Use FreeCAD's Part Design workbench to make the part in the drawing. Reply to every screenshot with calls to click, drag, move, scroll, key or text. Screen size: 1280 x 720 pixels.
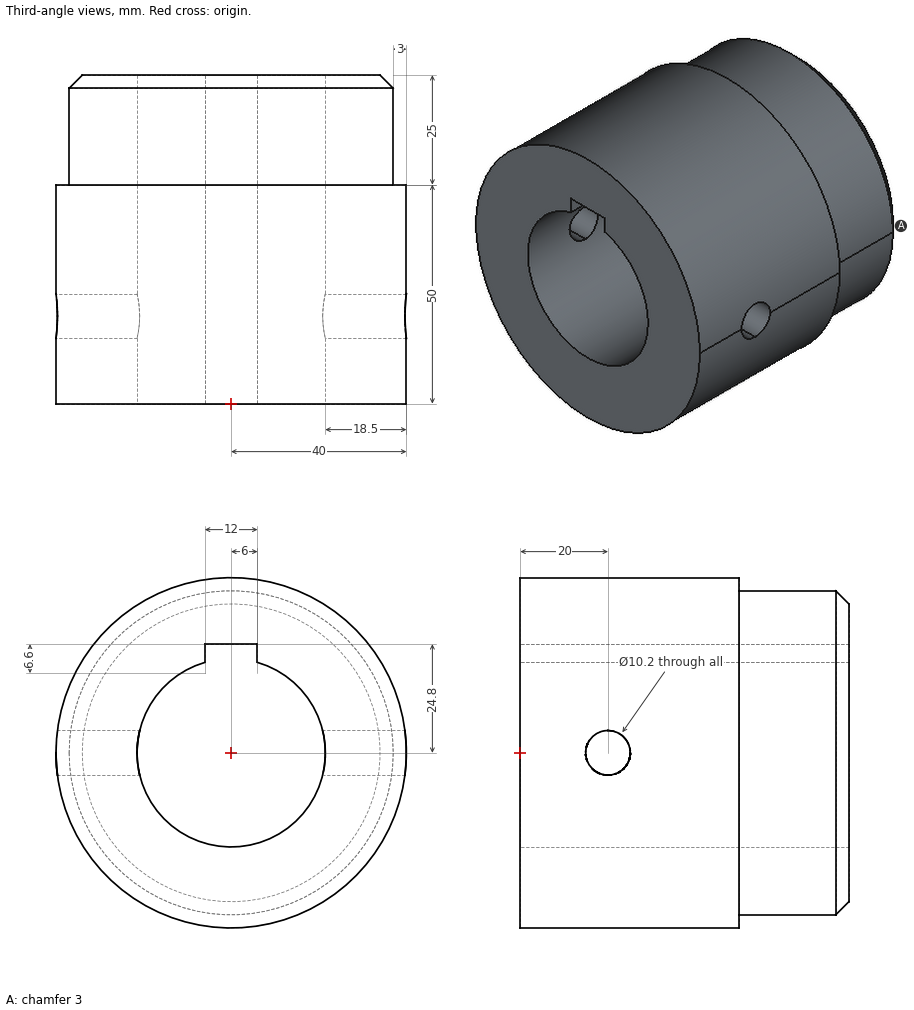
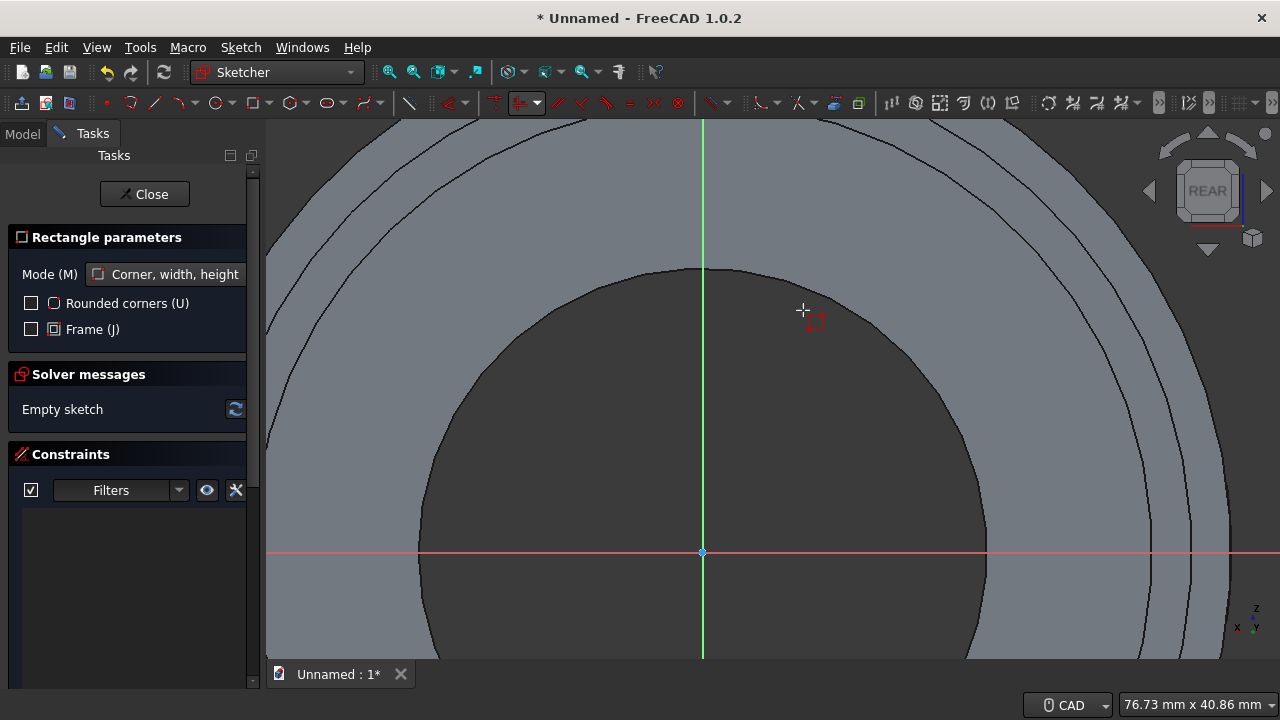
click(623, 225)
move(782, 312)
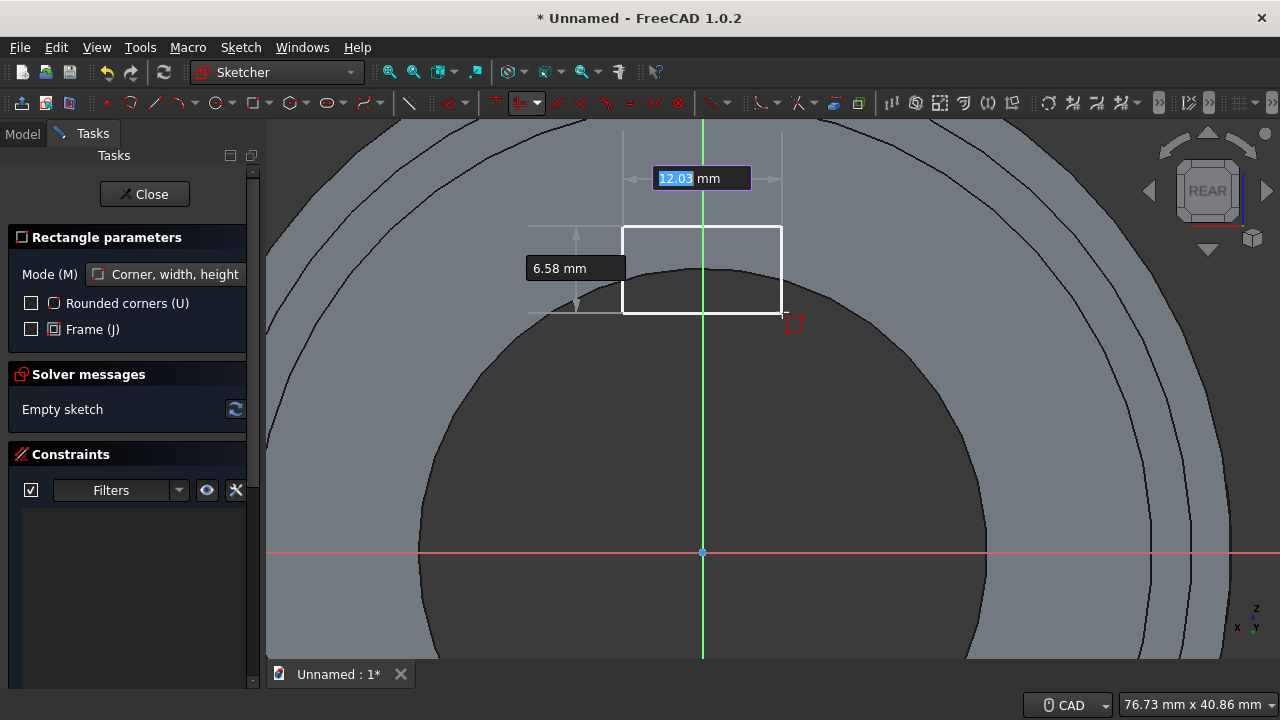
text(12)
key(Tab)
text(6.6)
key(Return)
key(Escape)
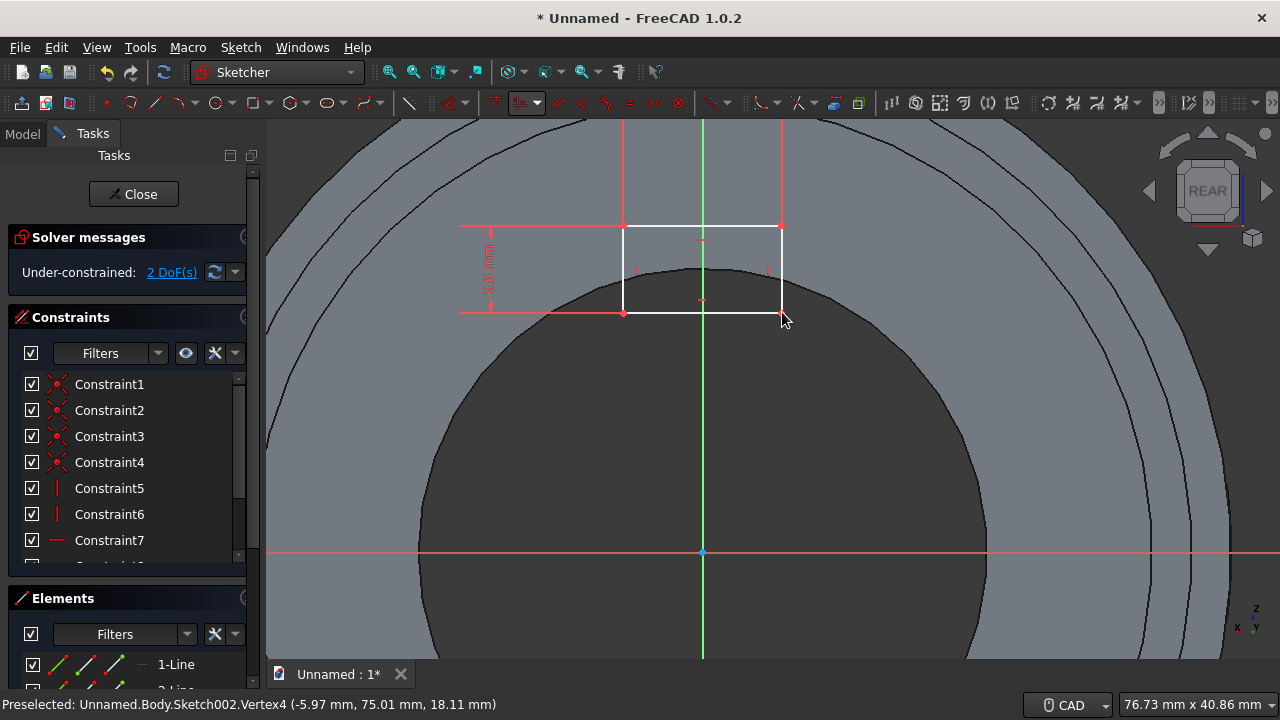
click(448, 104)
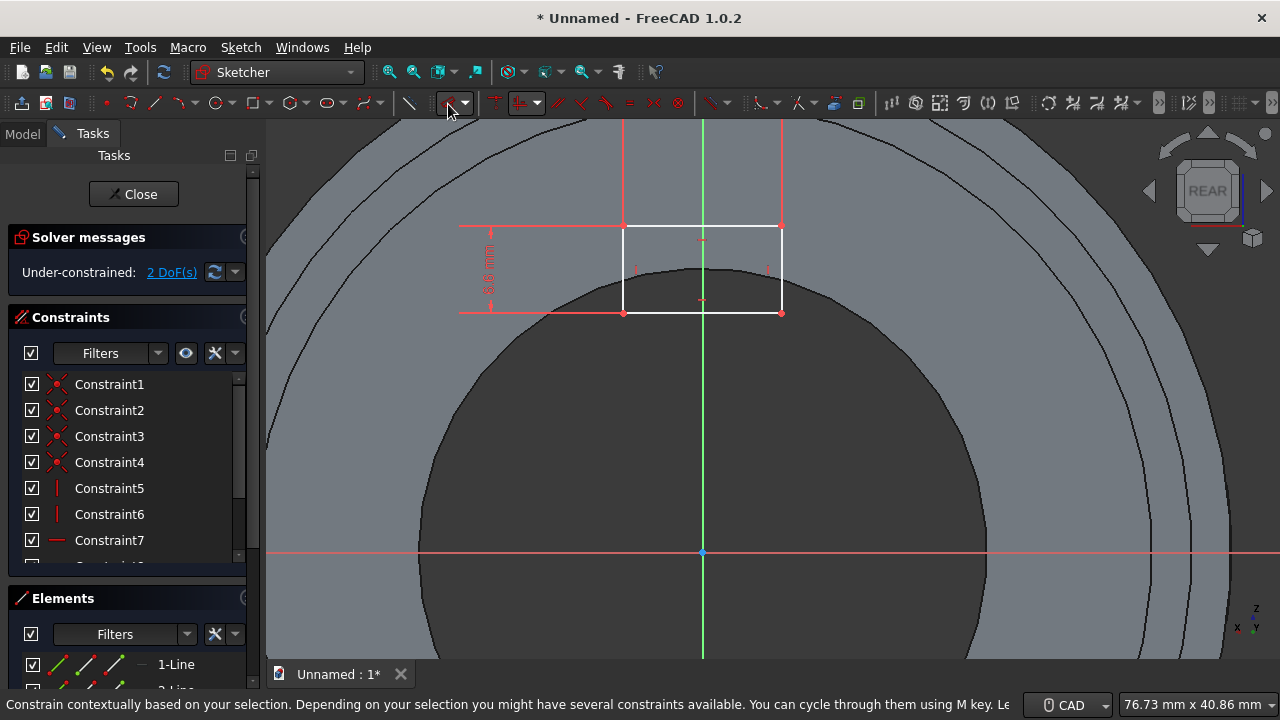
click(623, 226)
click(663, 587)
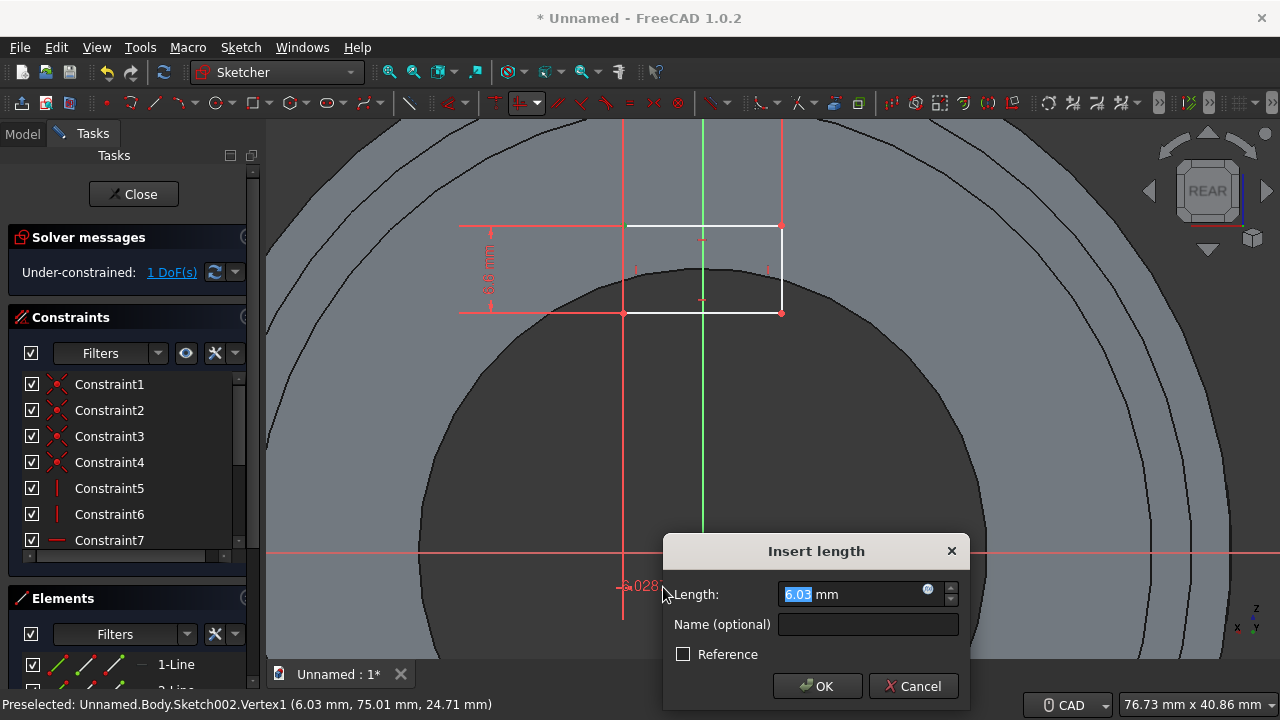
text(6)
key(Return)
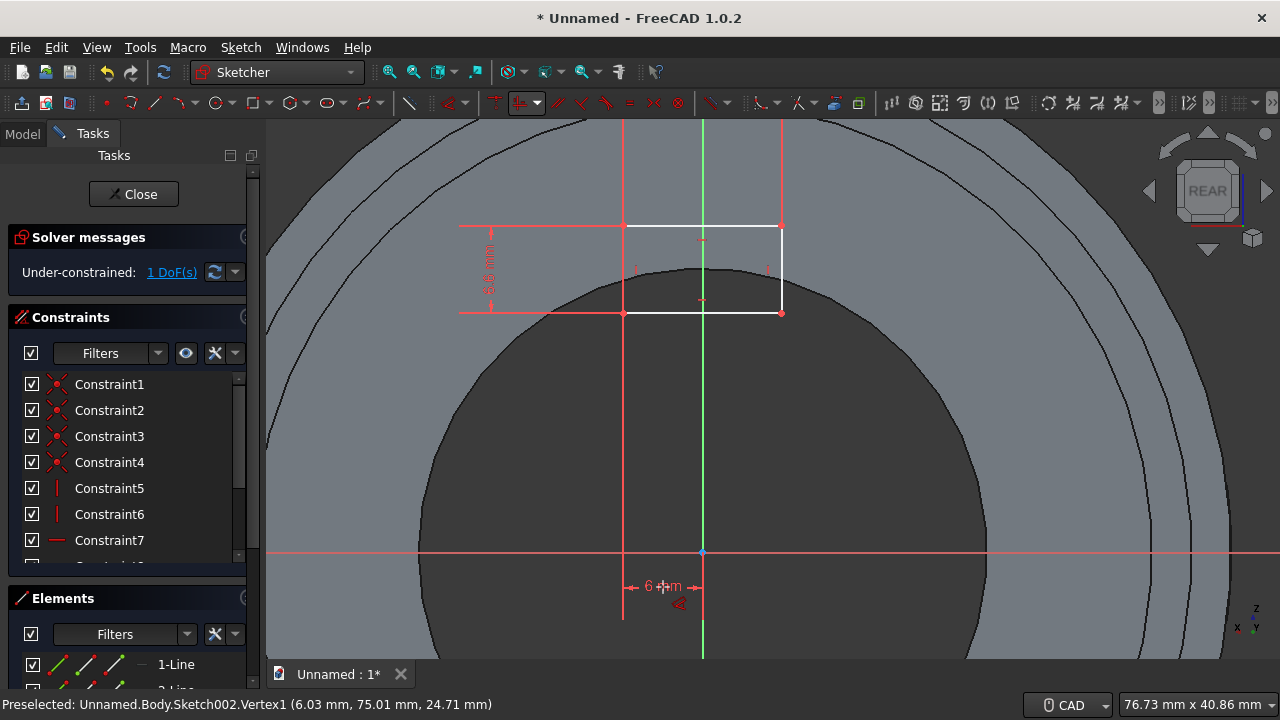
click(623, 226)
click(589, 389)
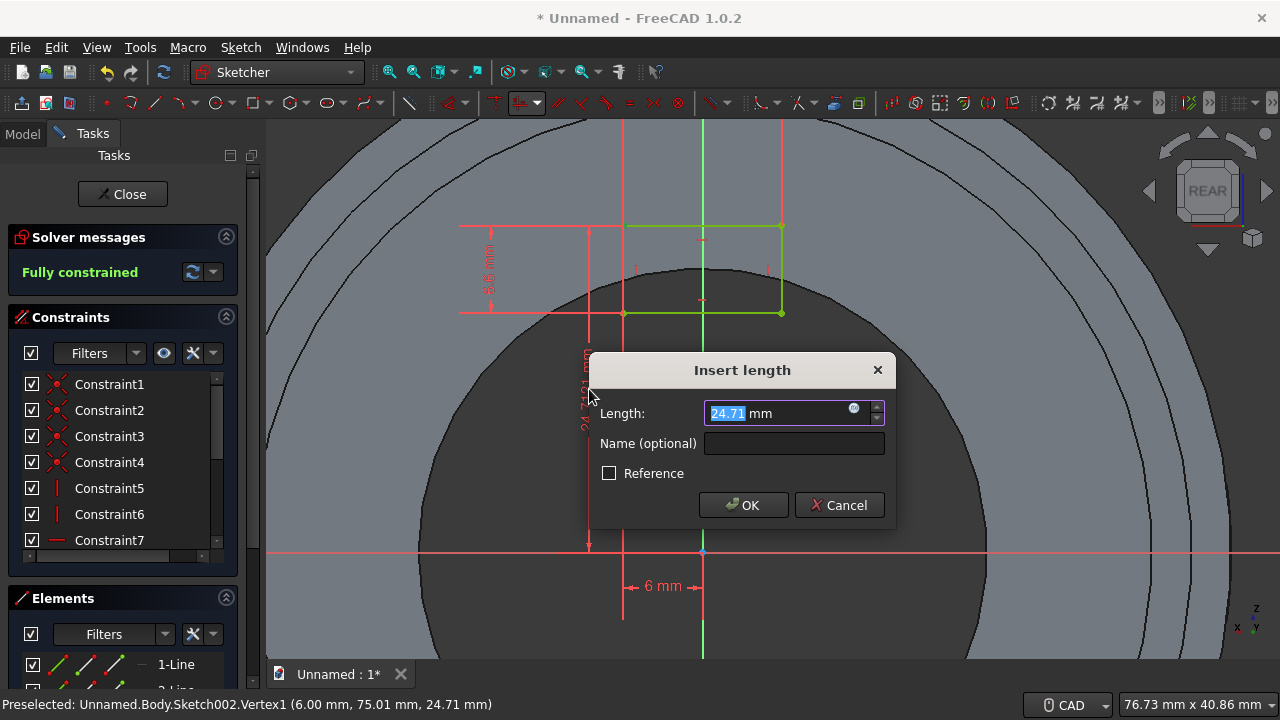
text(24.8)
key(Return)
key(Escape)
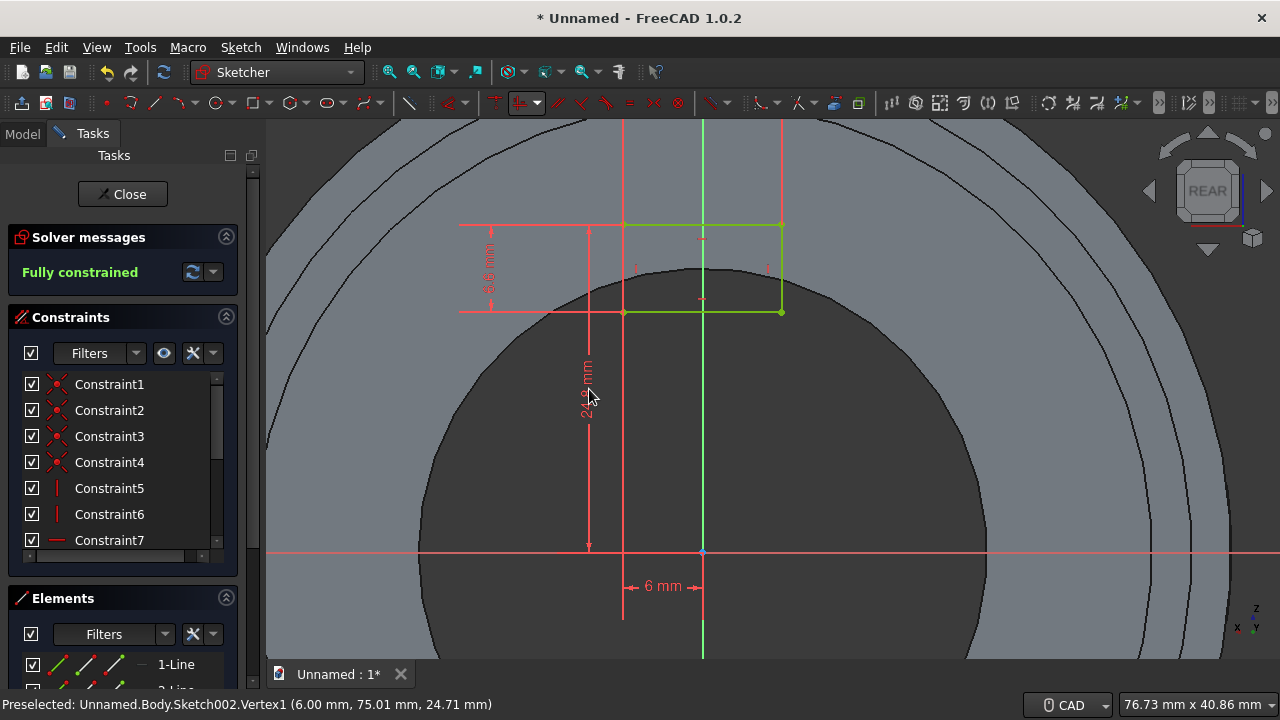
click(123, 194)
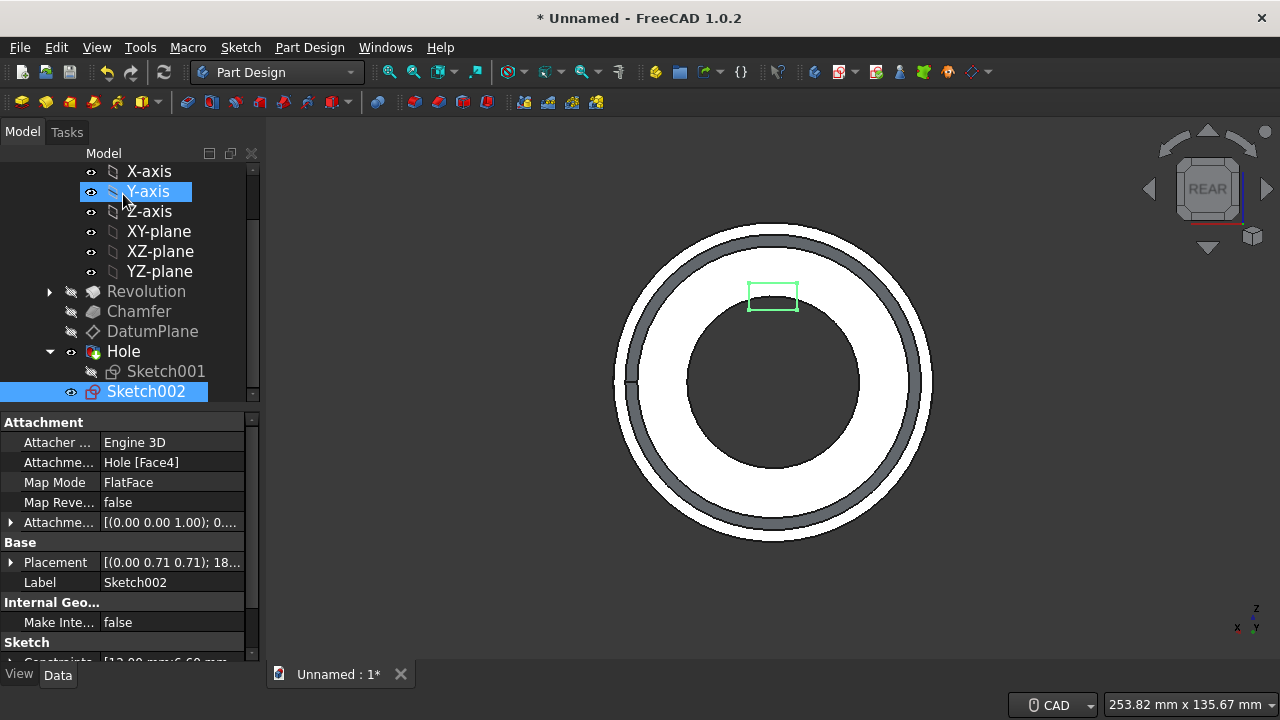
click(188, 102)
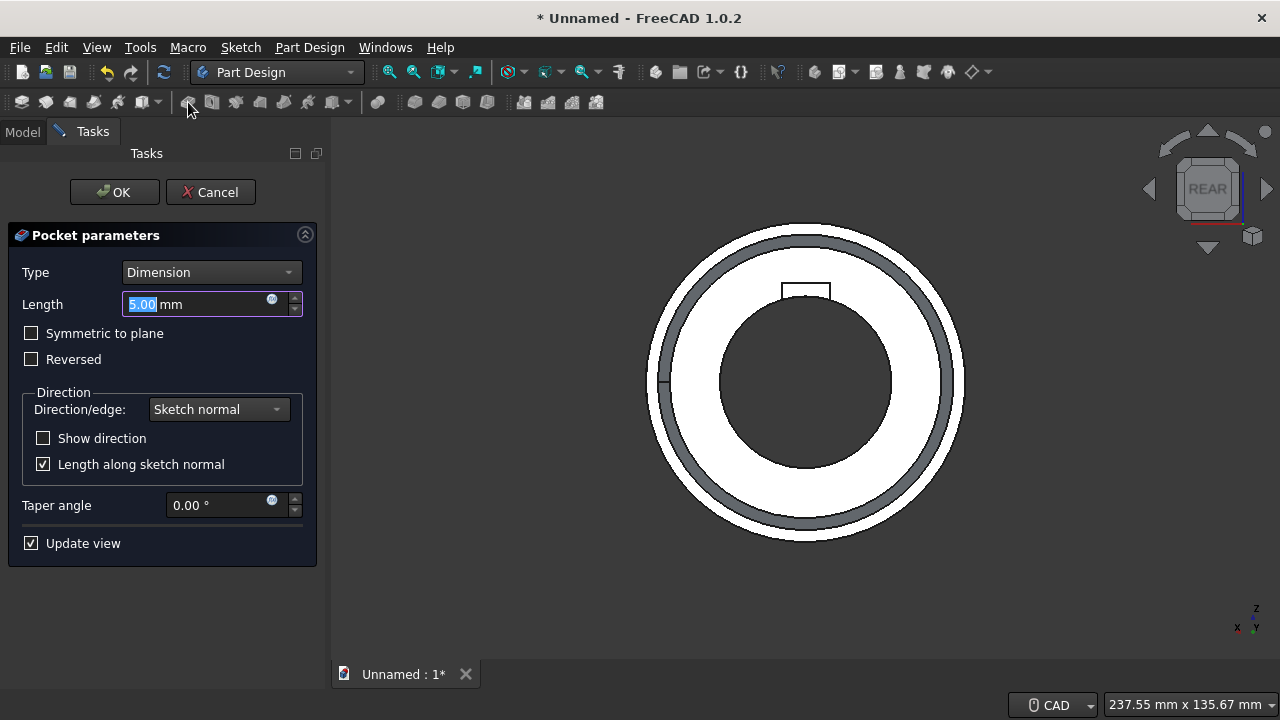
click(212, 272)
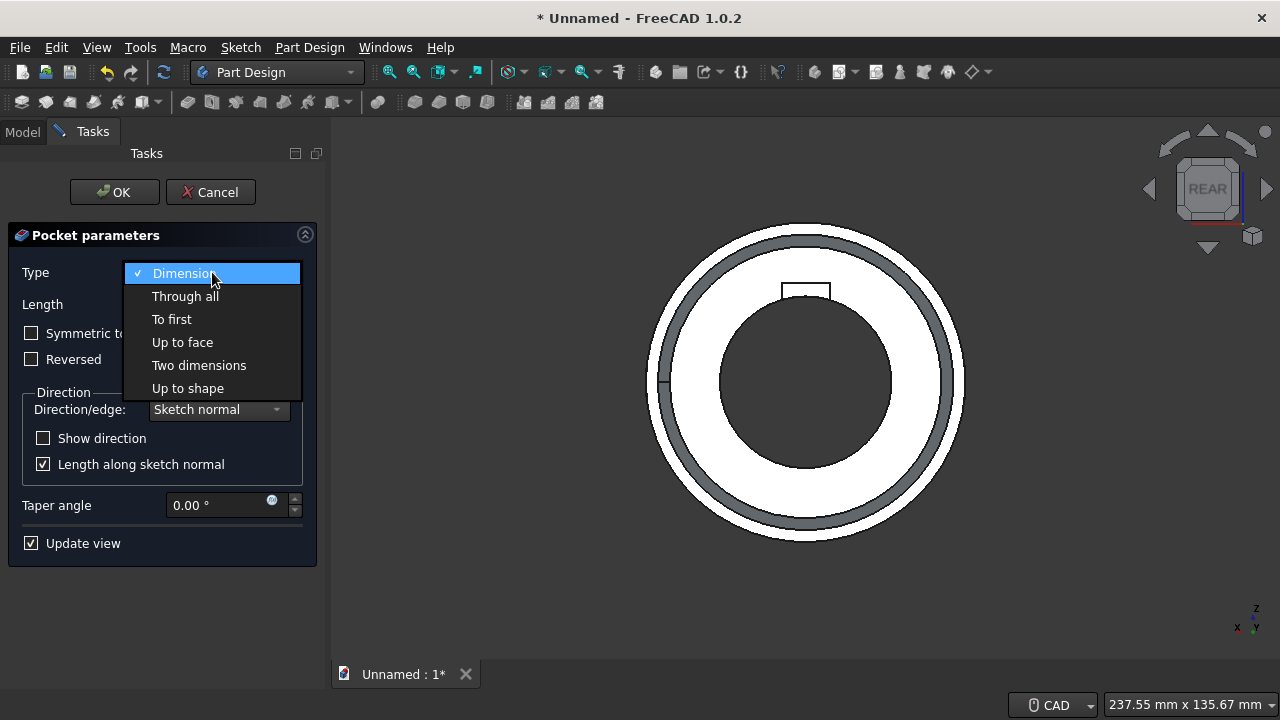
click(212, 320)